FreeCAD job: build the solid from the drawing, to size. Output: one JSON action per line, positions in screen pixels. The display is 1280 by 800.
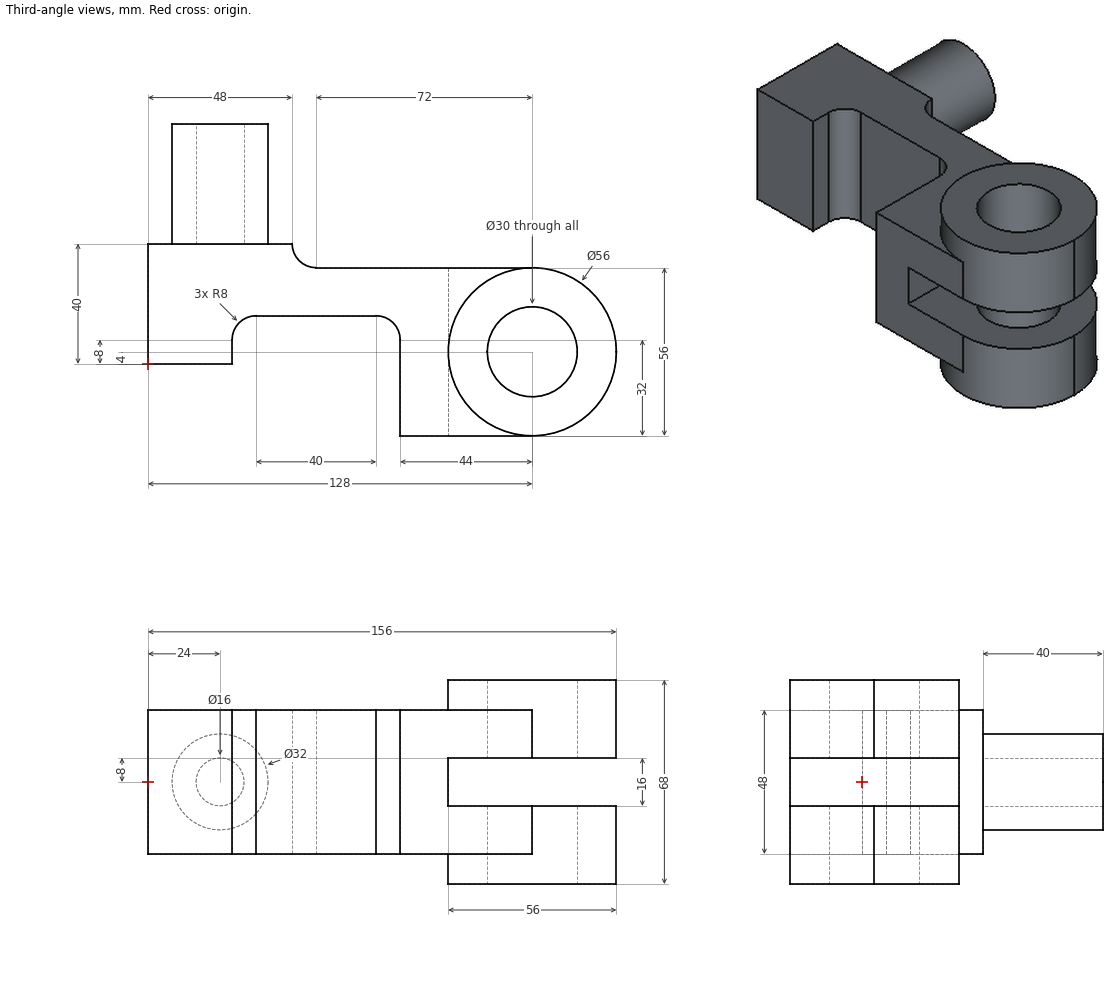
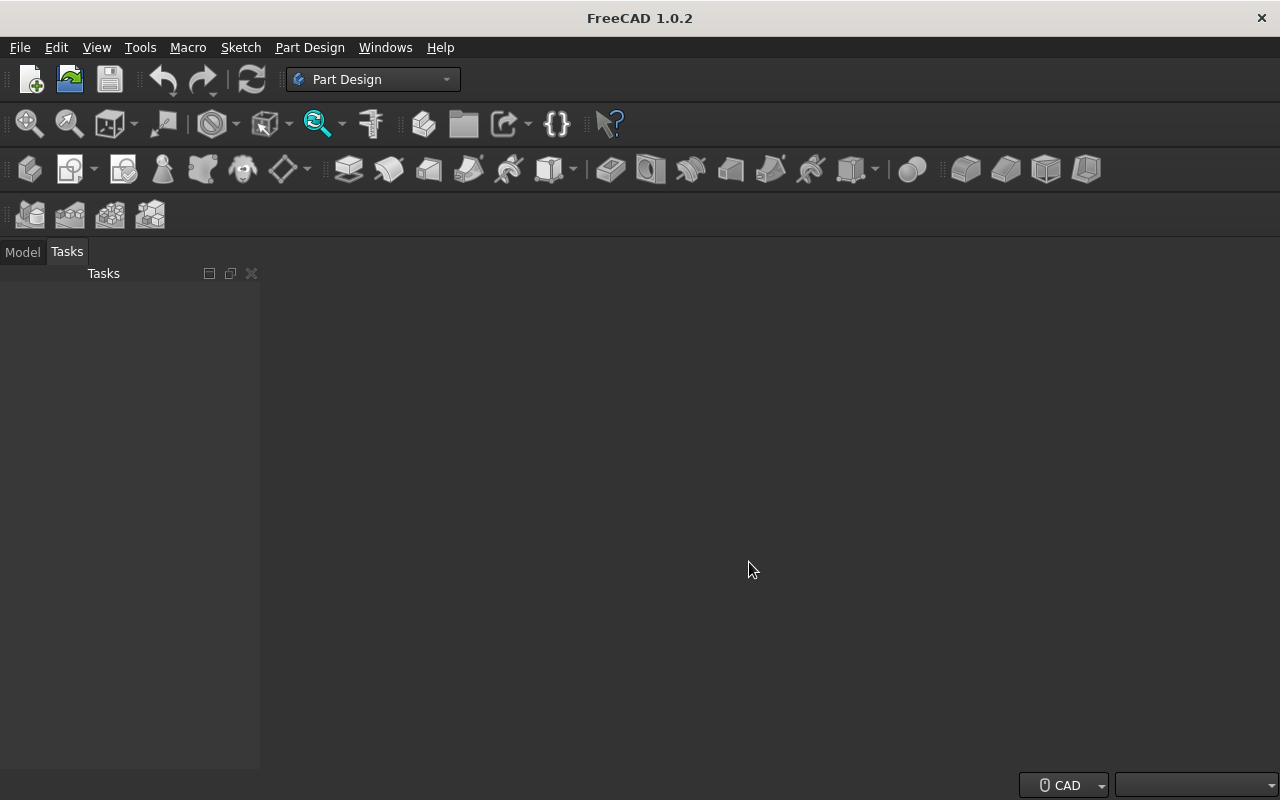
{"action": "left_click", "coordinate": [30, 80]}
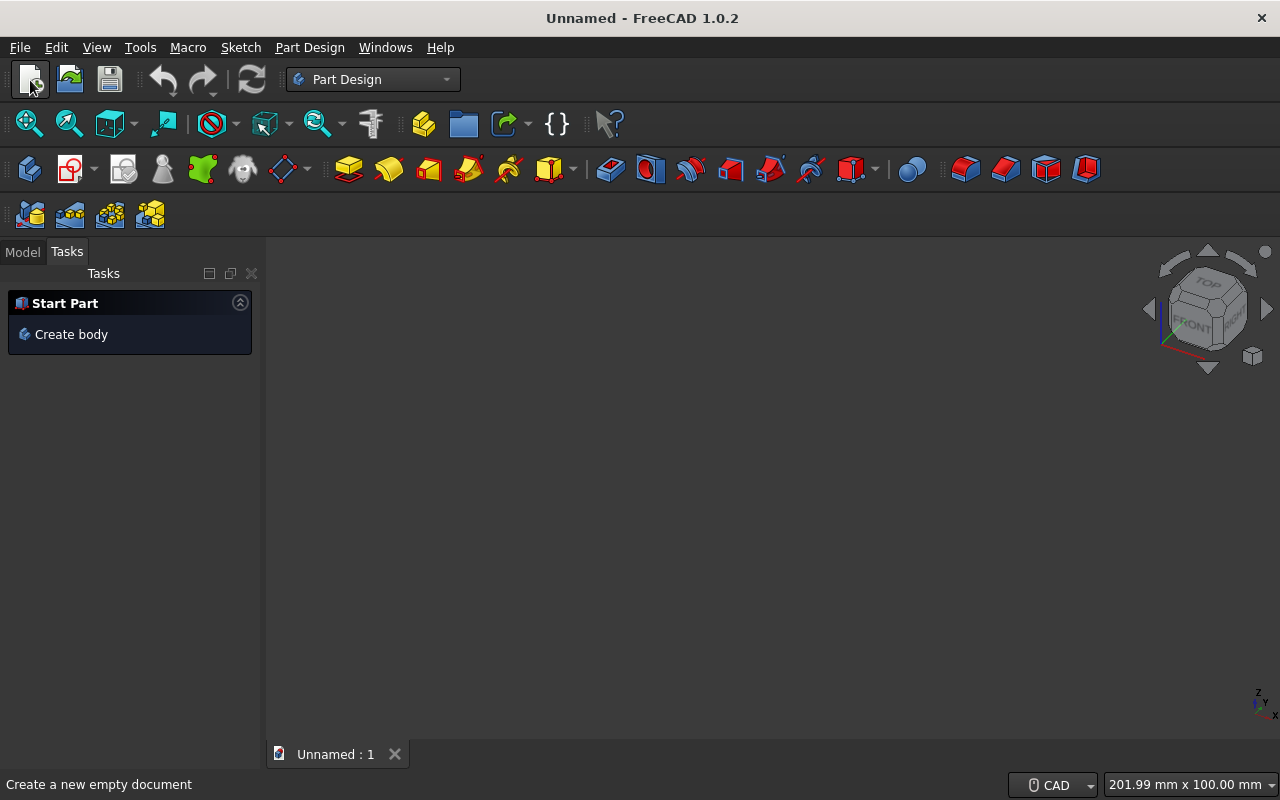
{"action": "left_click", "coordinate": [70, 170]}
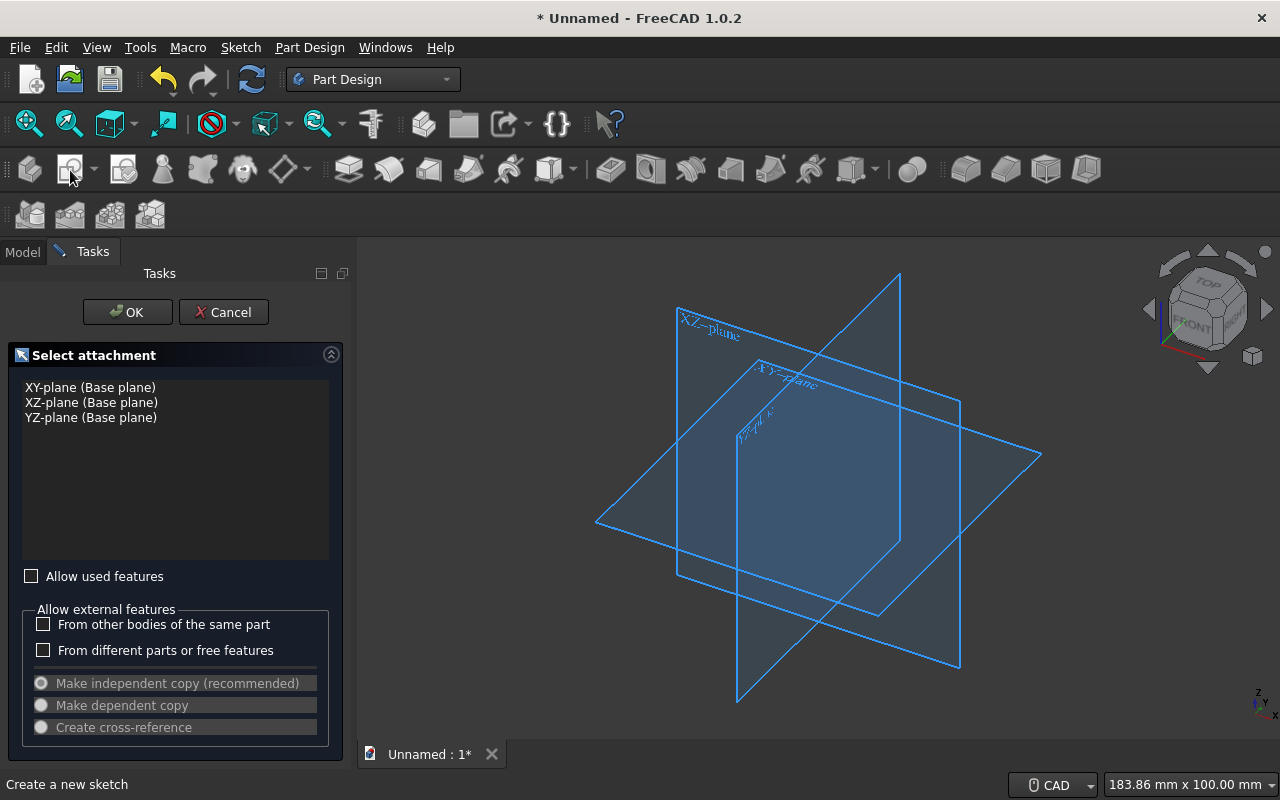
{"action": "left_click", "coordinate": [82, 388]}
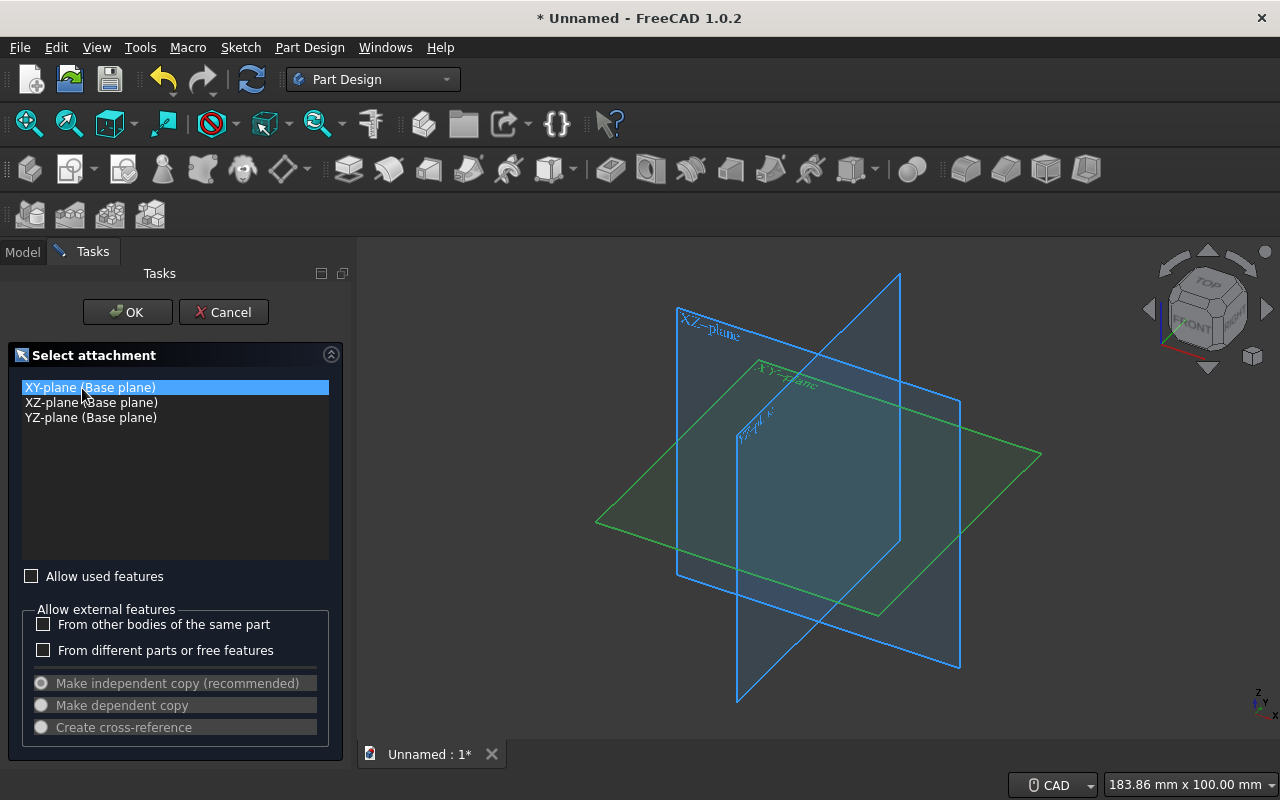
{"action": "left_click", "coordinate": [128, 312]}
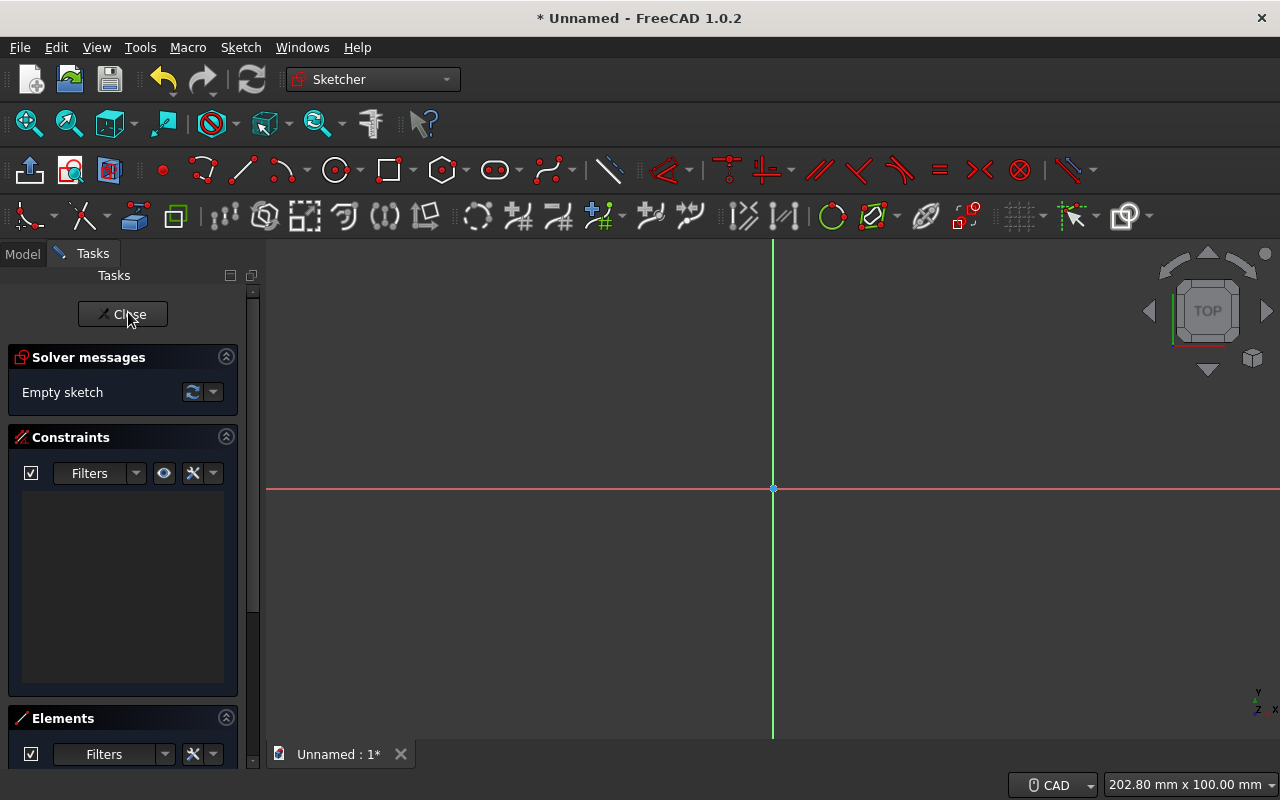
{"action": "scroll", "coordinate": [294, 570], "scroll_direction": "down", "scroll_amount": 2}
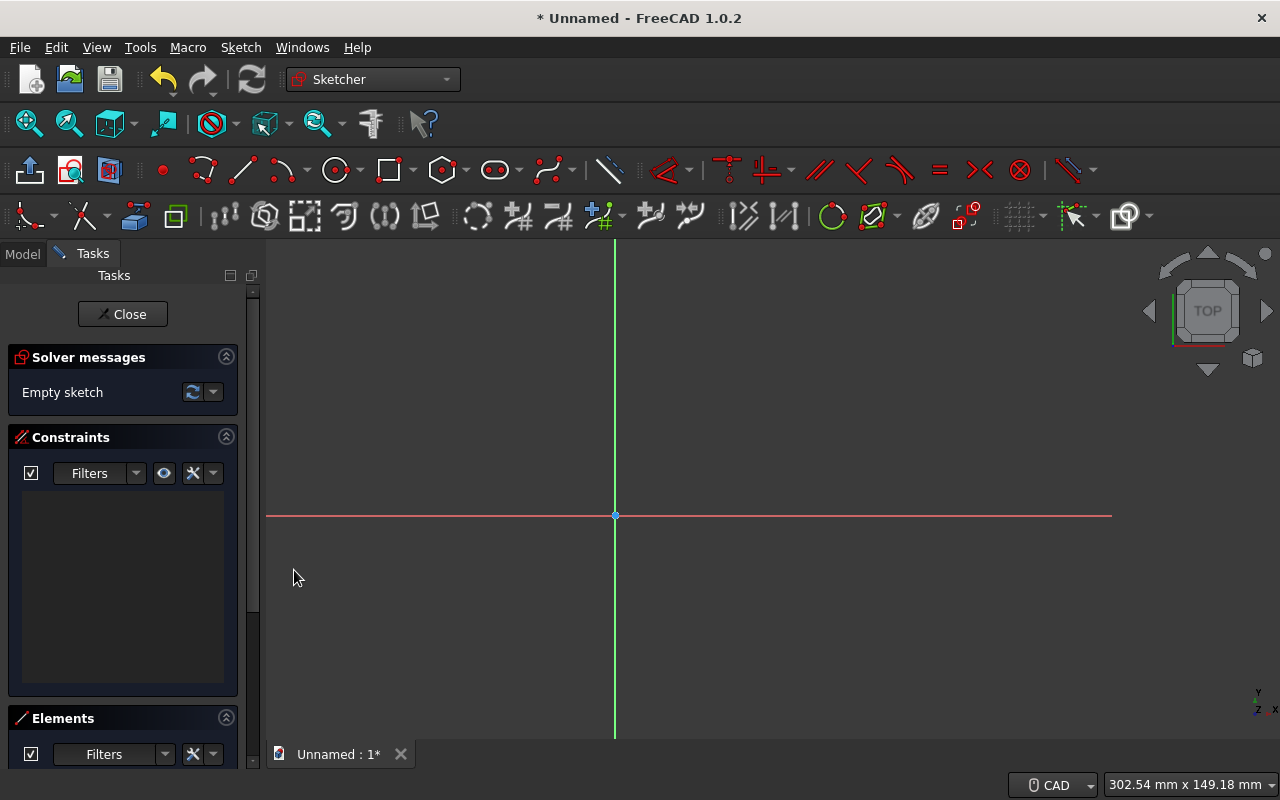
{"action": "scroll", "coordinate": [1084, 489], "scroll_direction": "up", "scroll_amount": 2}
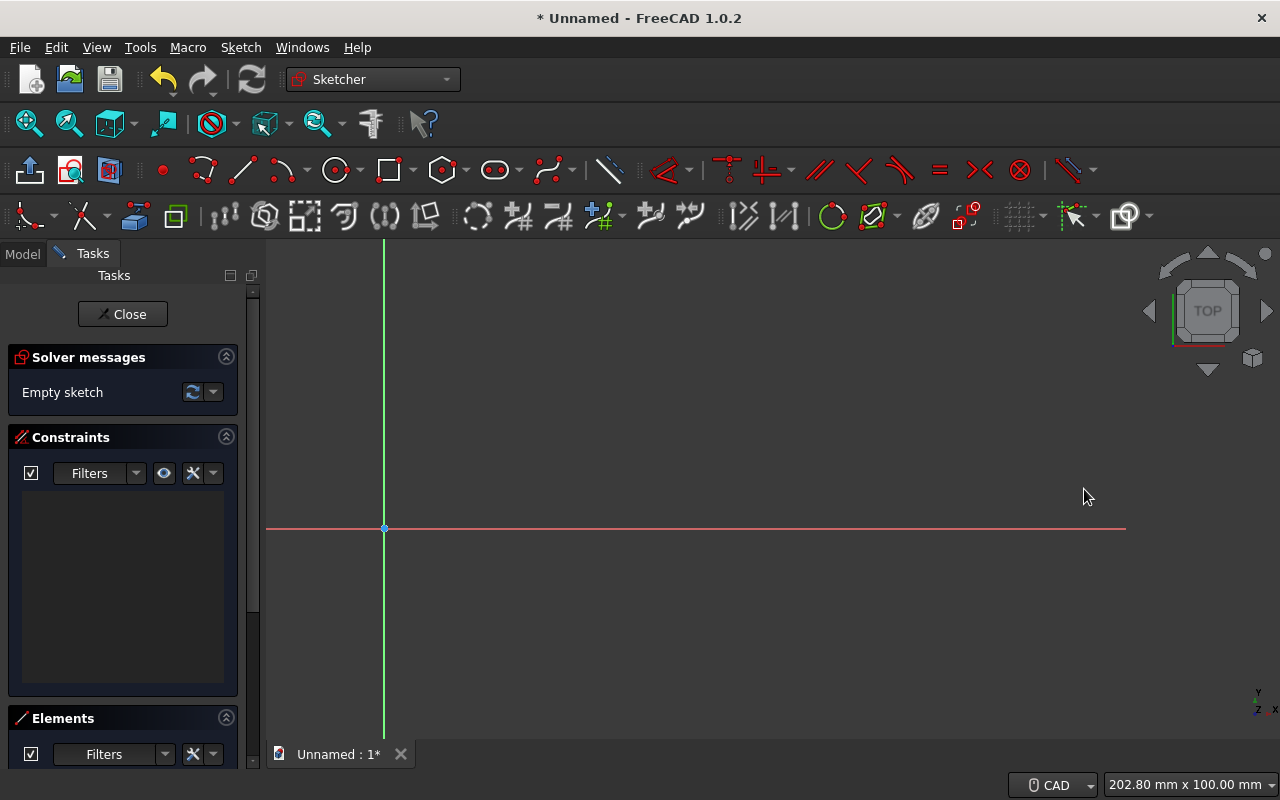
{"action": "key", "text": "g l"}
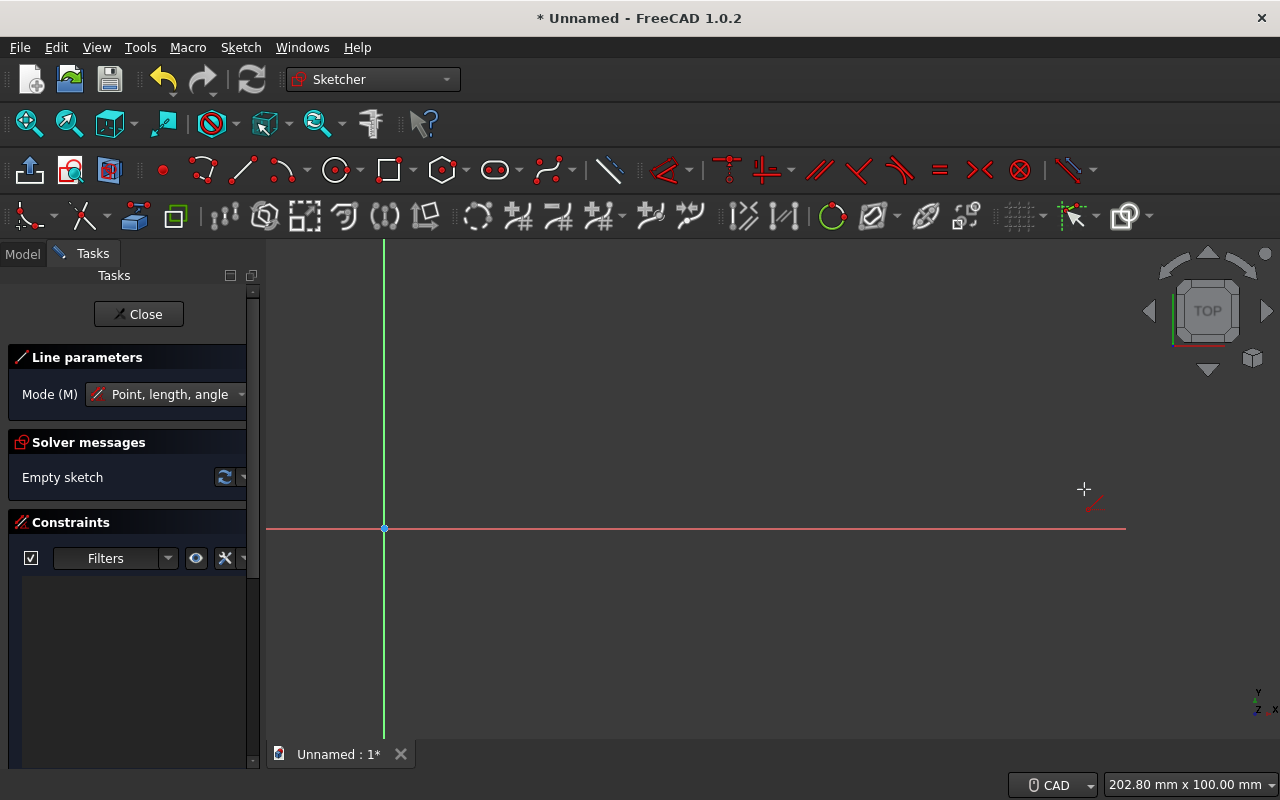
{"action": "left_click", "coordinate": [564, 449]}
{"action": "left_click", "coordinate": [764, 449]}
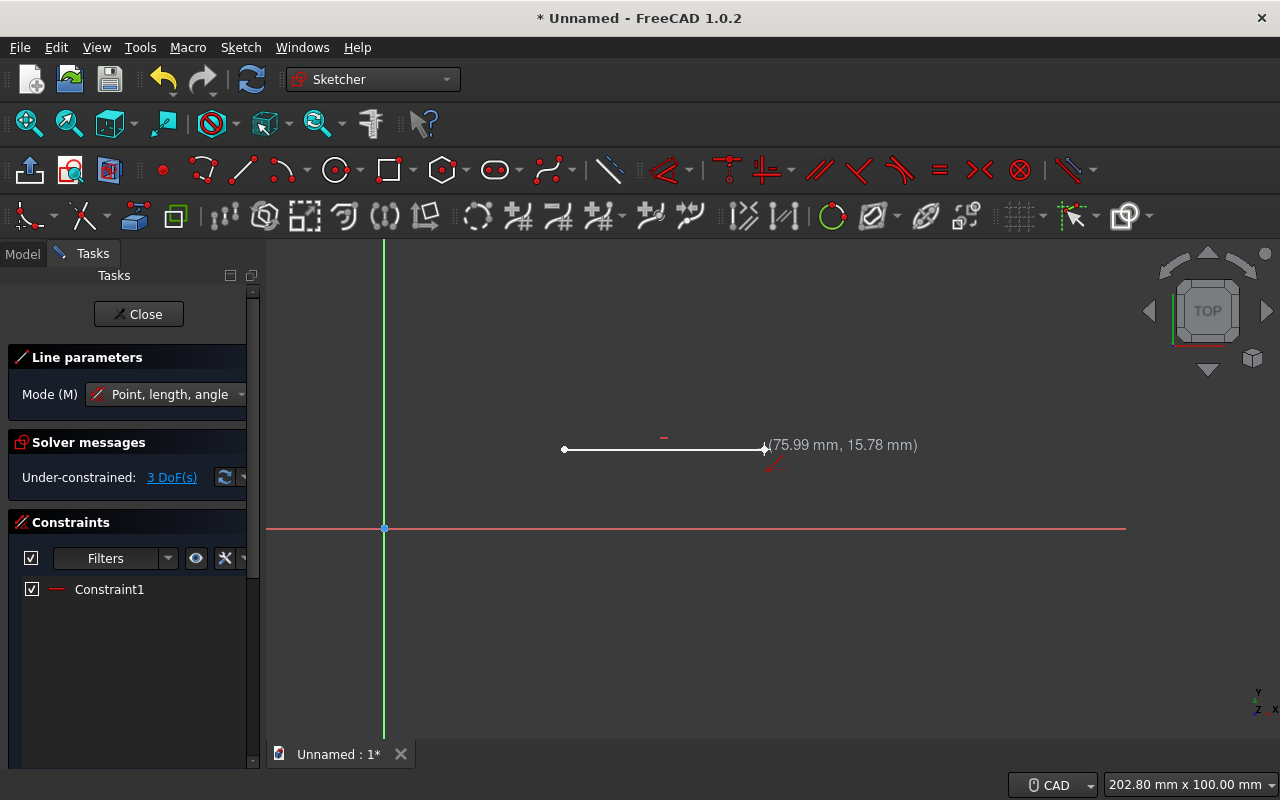
{"action": "key", "text": "g m"}